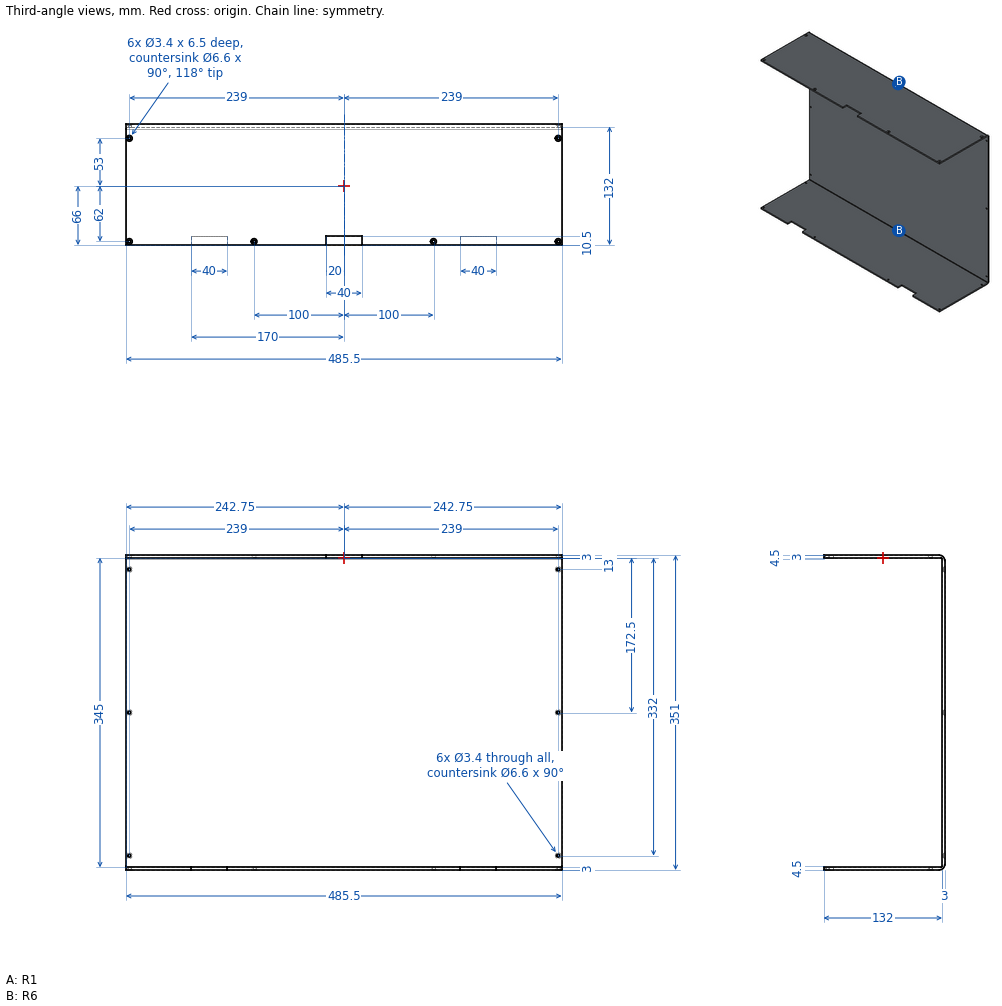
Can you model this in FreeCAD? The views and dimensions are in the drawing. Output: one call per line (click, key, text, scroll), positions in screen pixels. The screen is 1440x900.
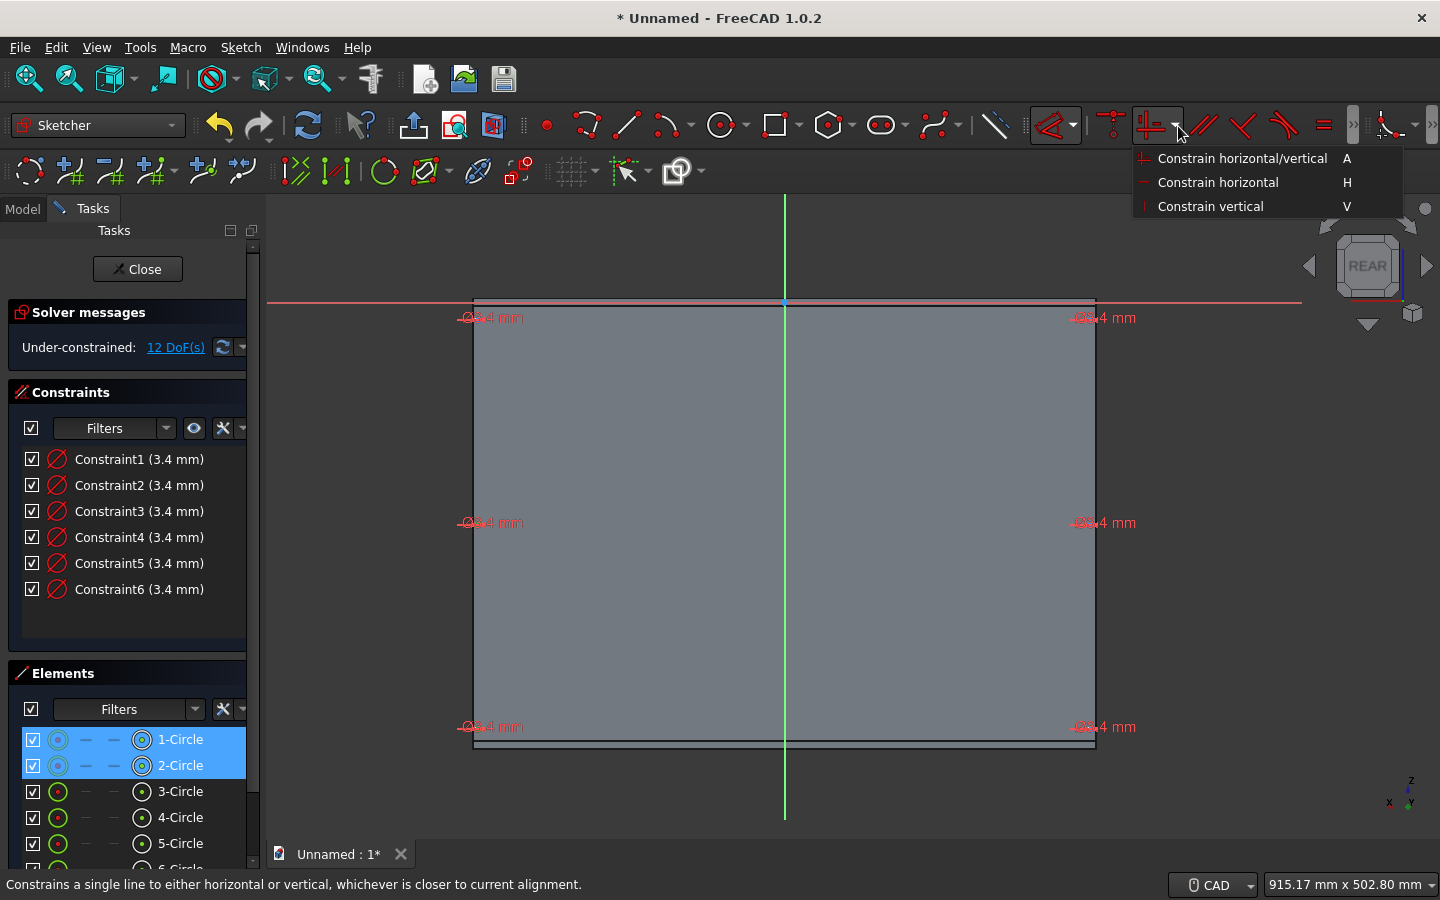
click(1268, 206)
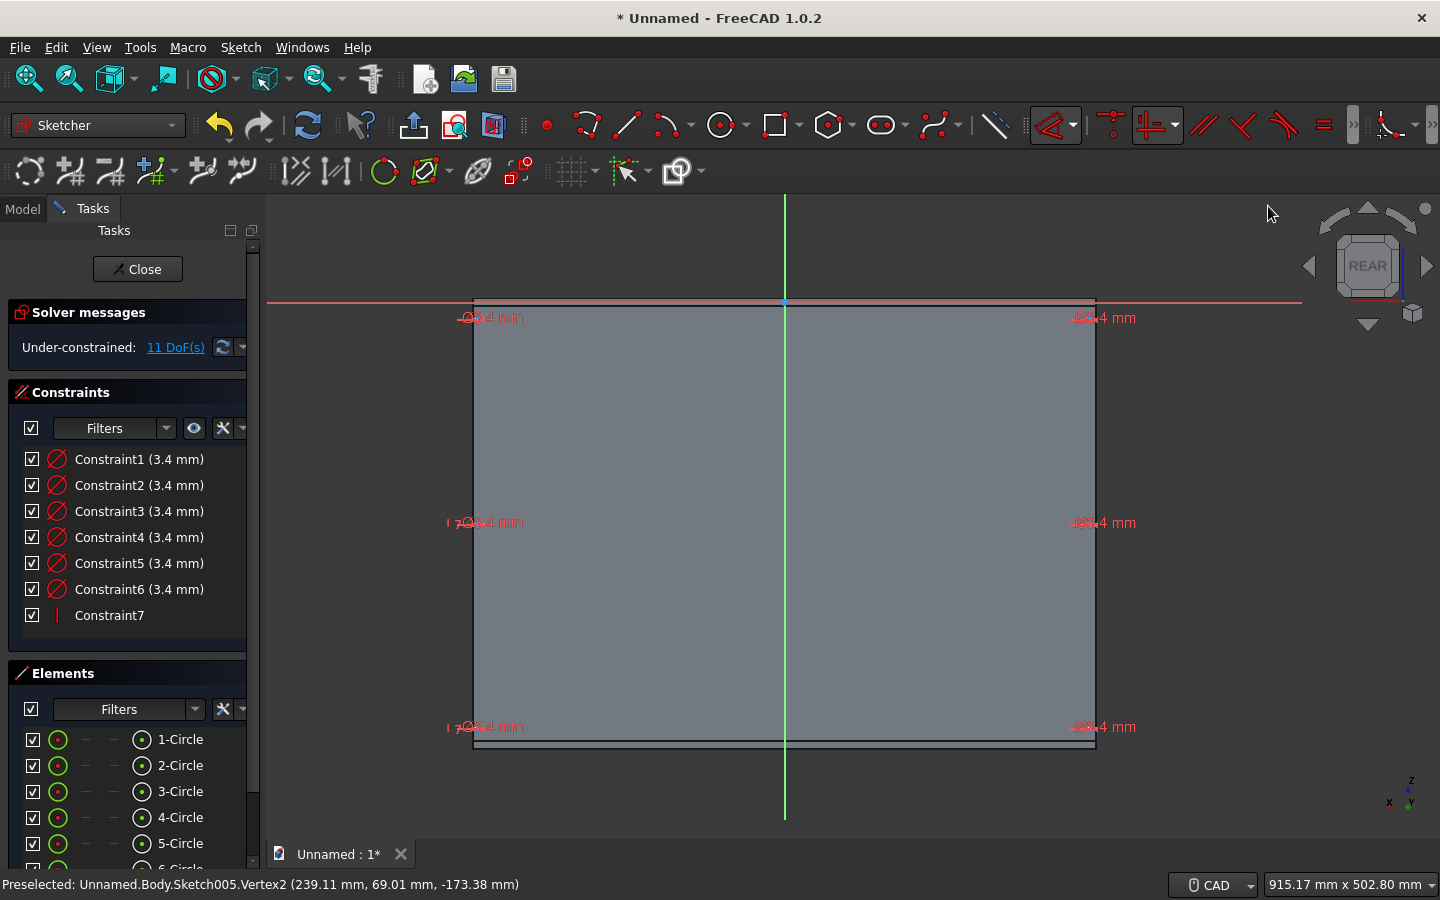
click(478, 525)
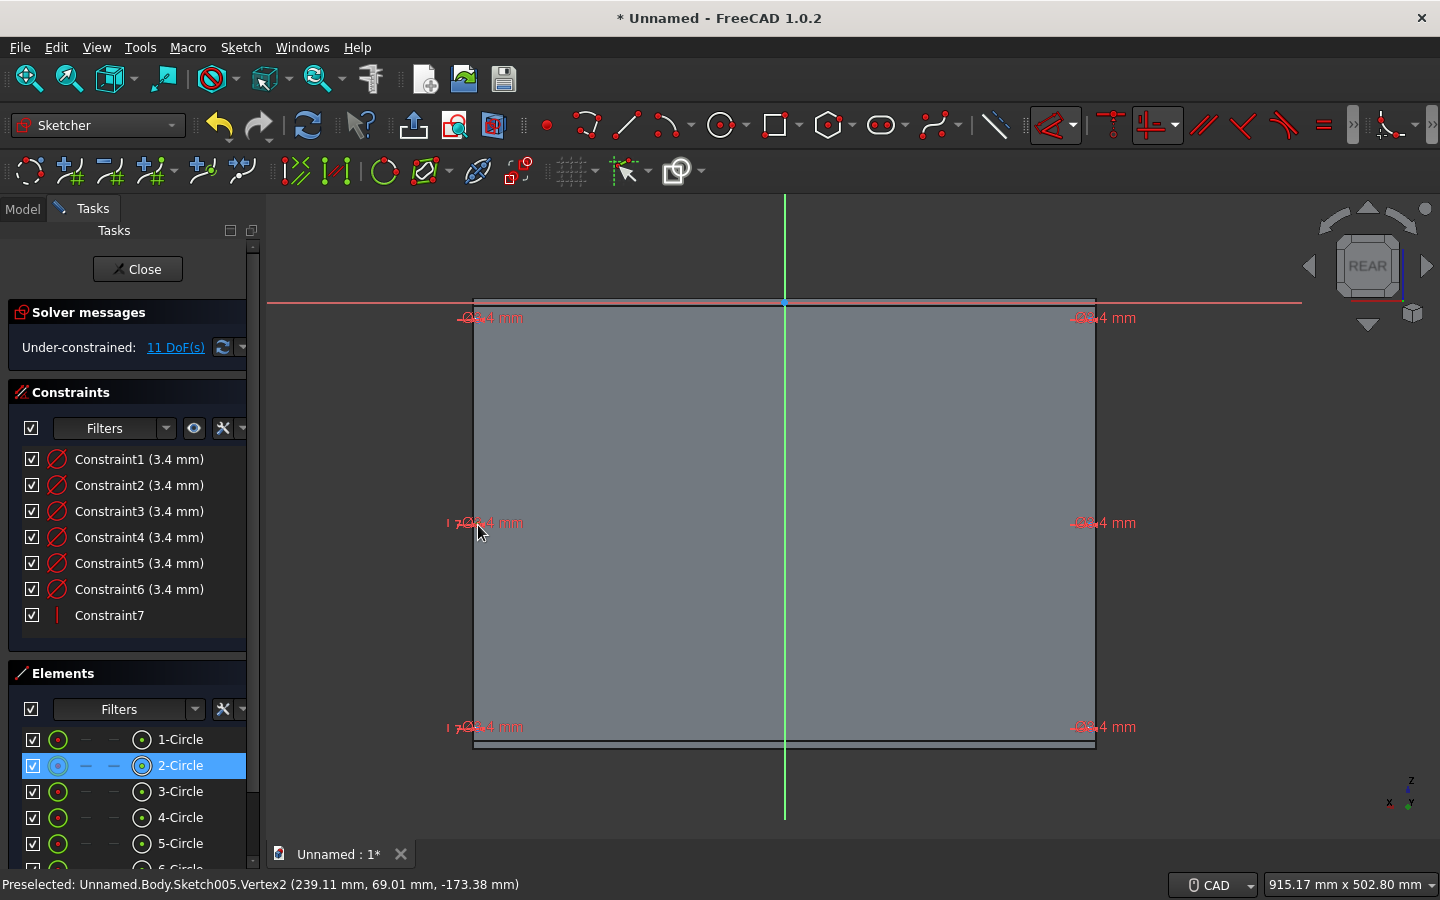
click(478, 320)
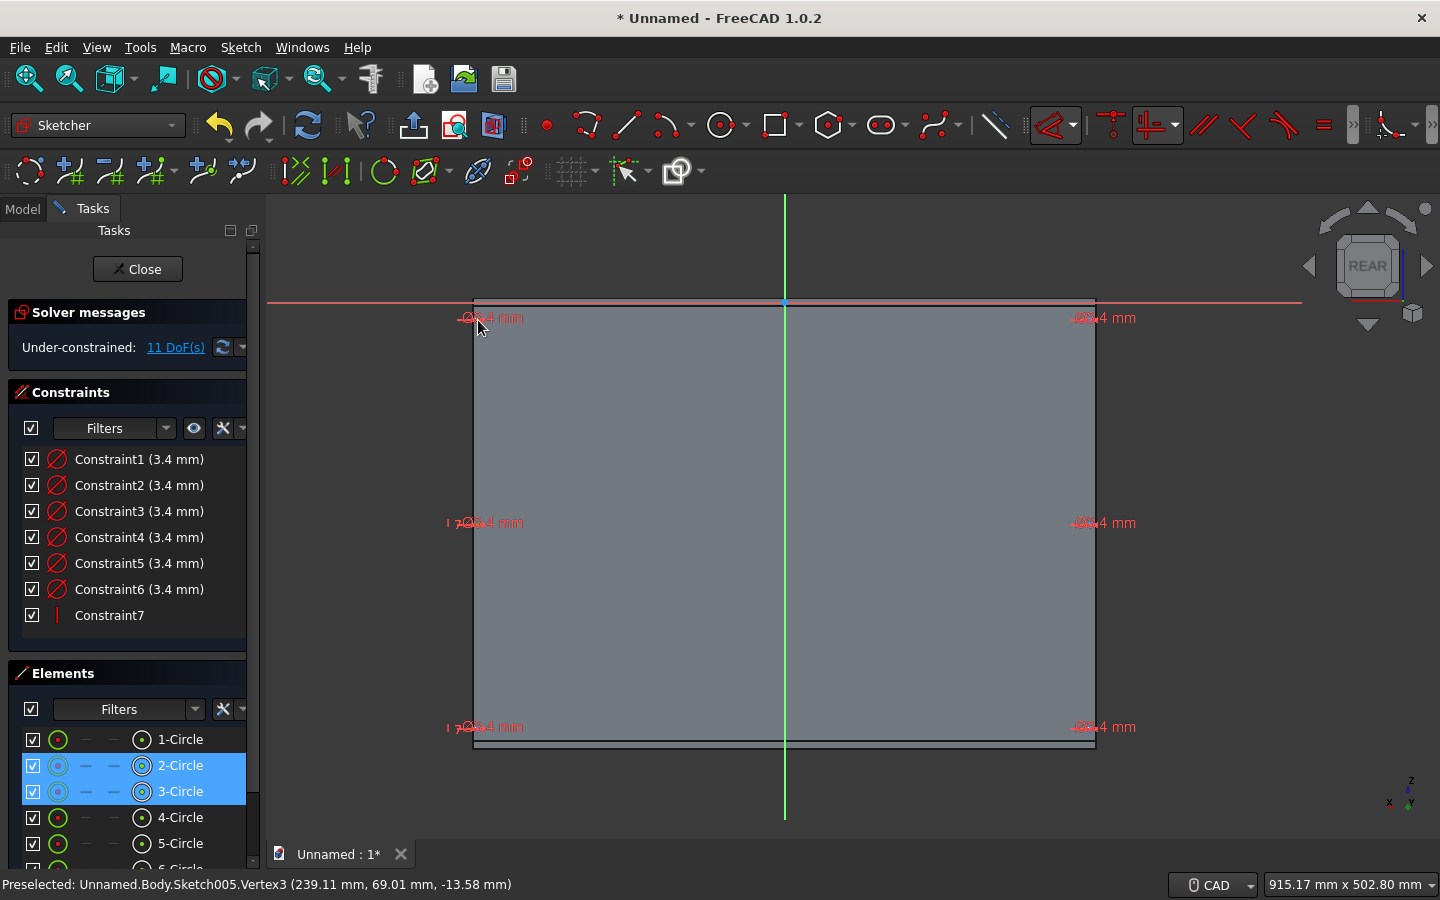
key(v)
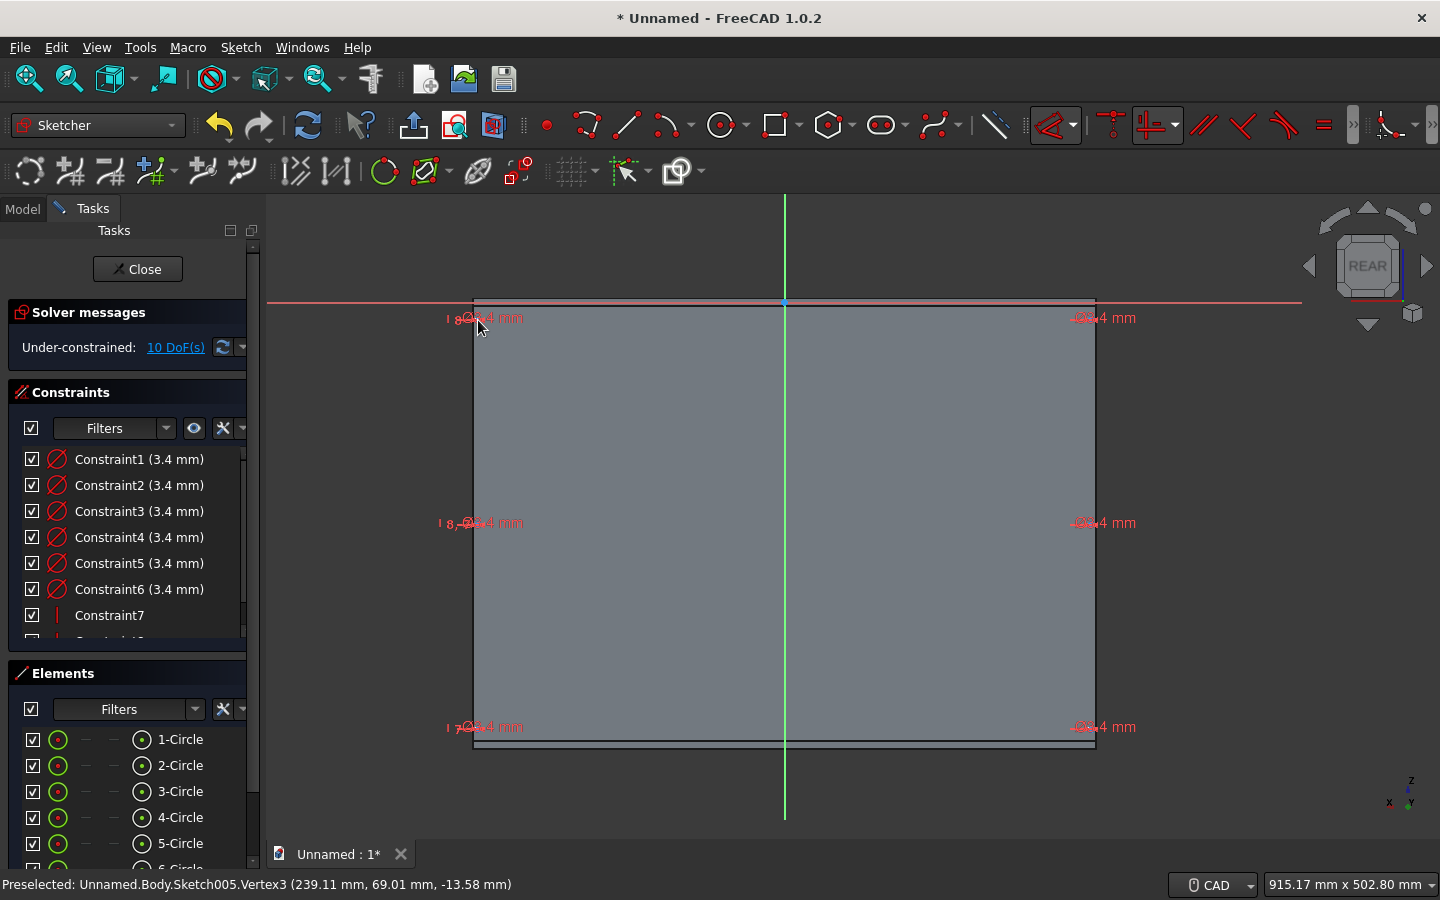
click(478, 729)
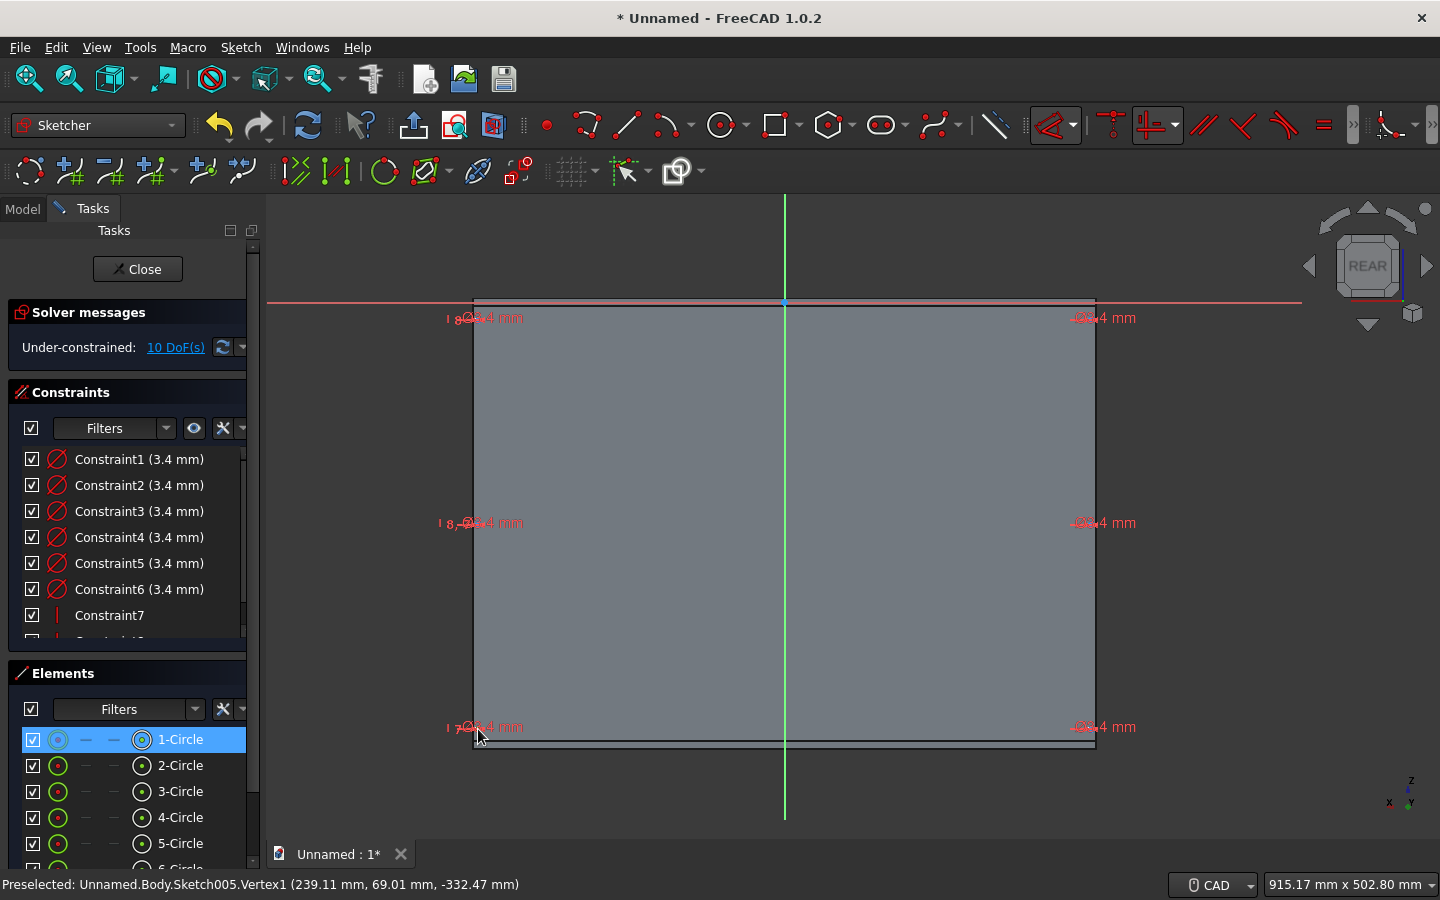
click(1091, 729)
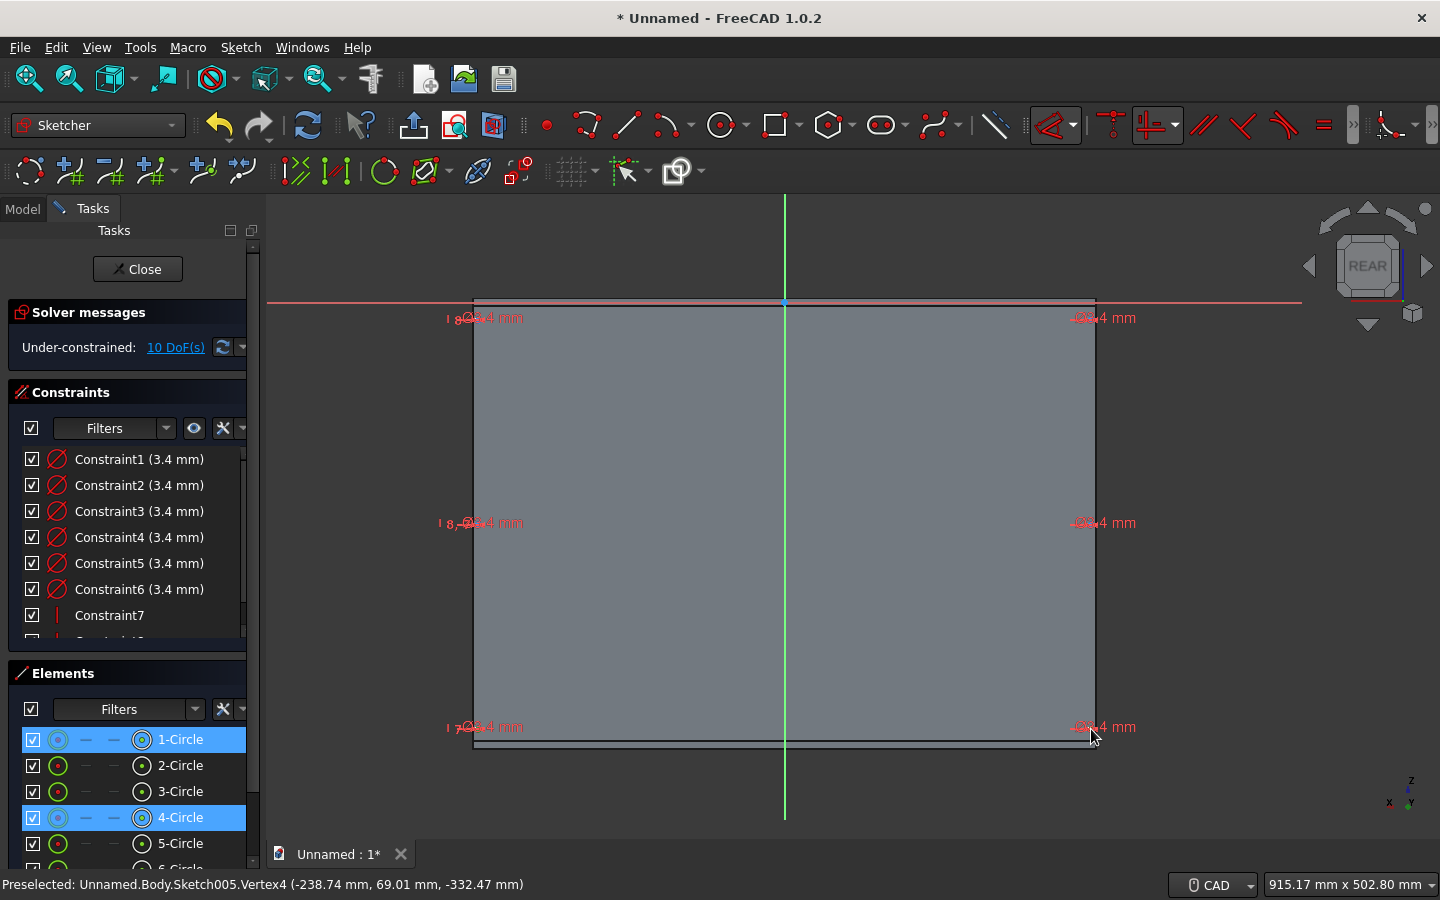
key(h)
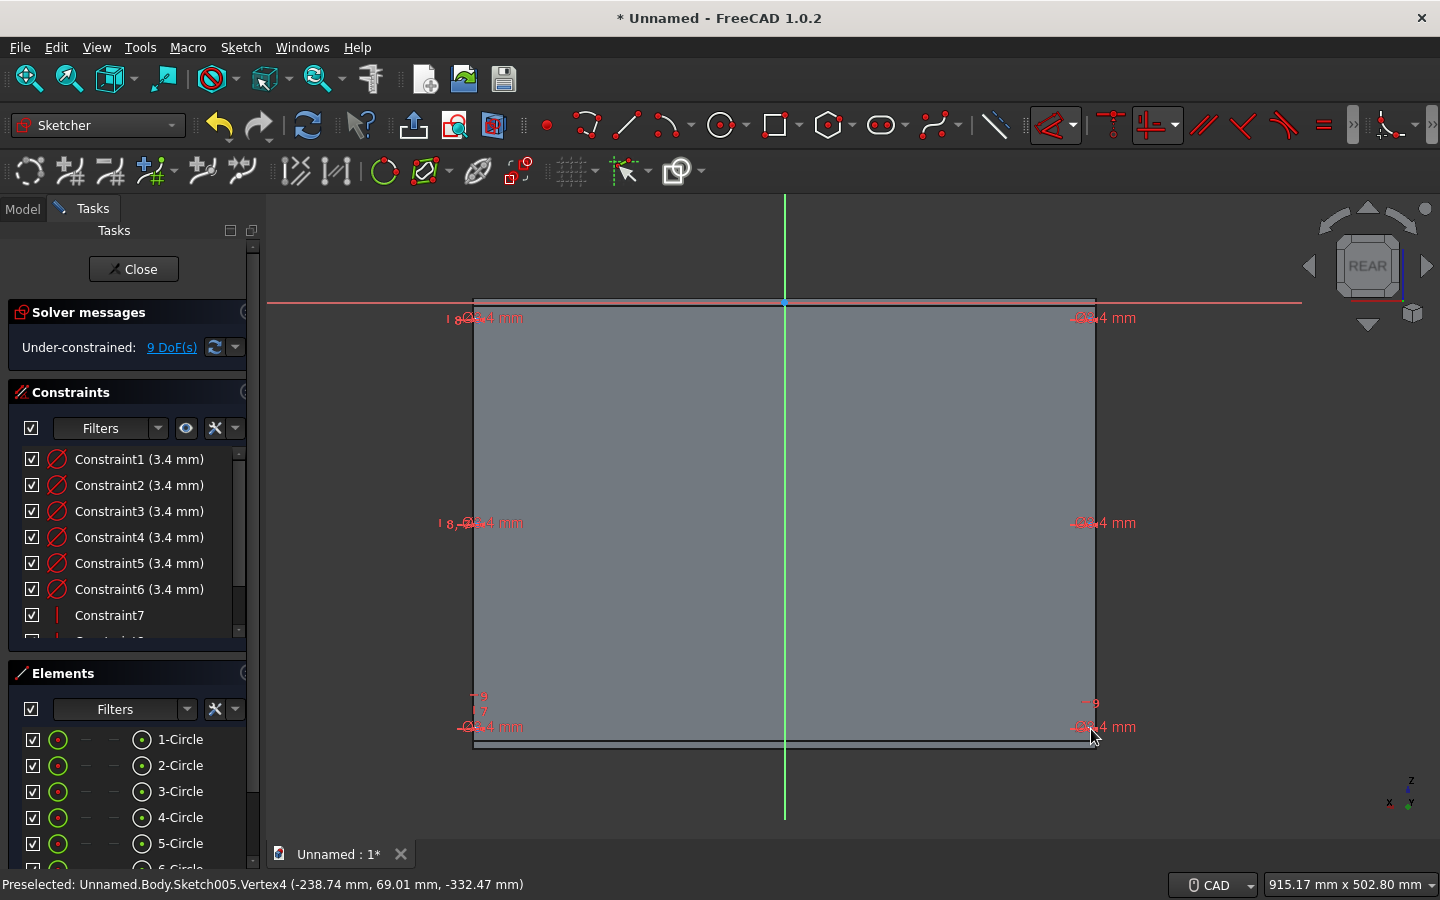
click(1091, 729)